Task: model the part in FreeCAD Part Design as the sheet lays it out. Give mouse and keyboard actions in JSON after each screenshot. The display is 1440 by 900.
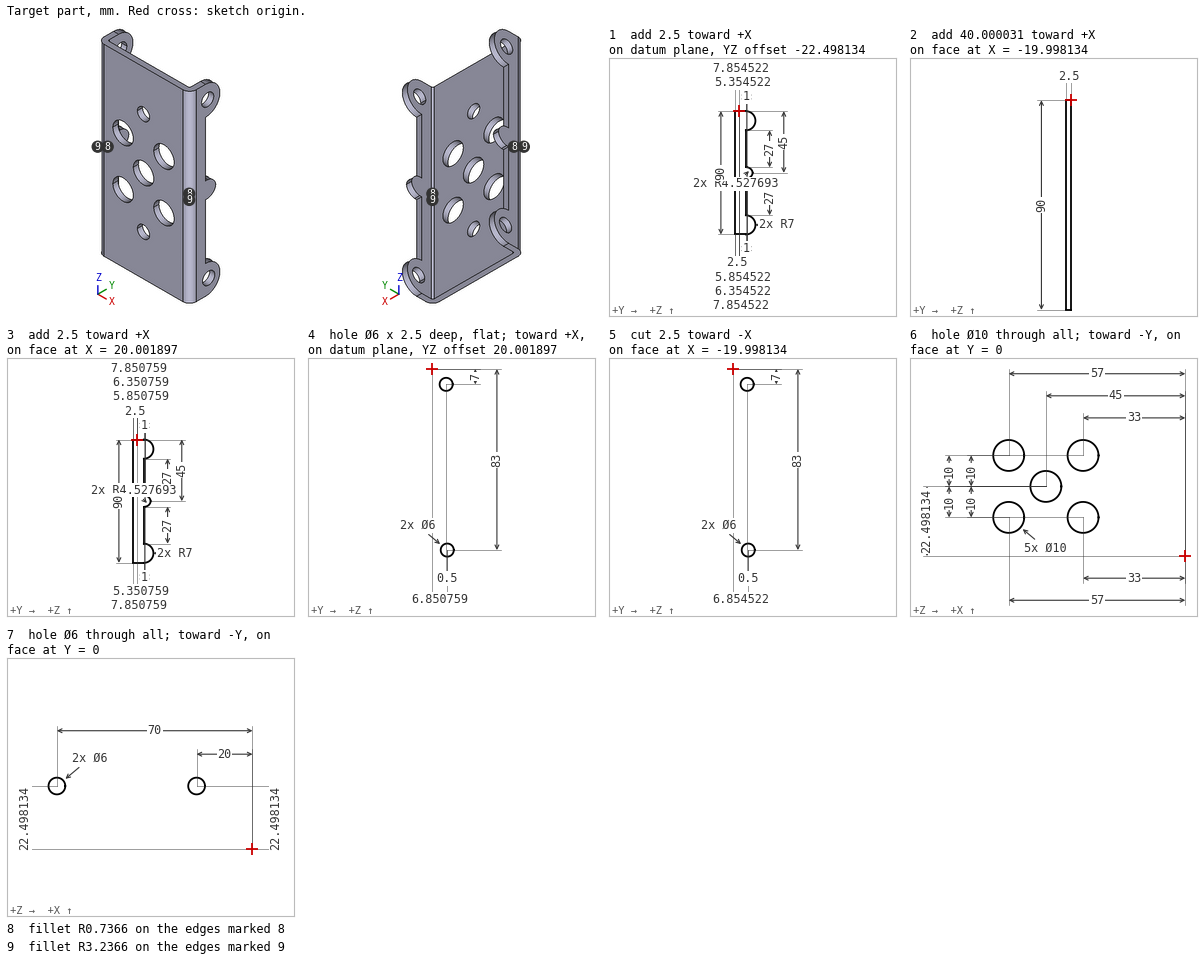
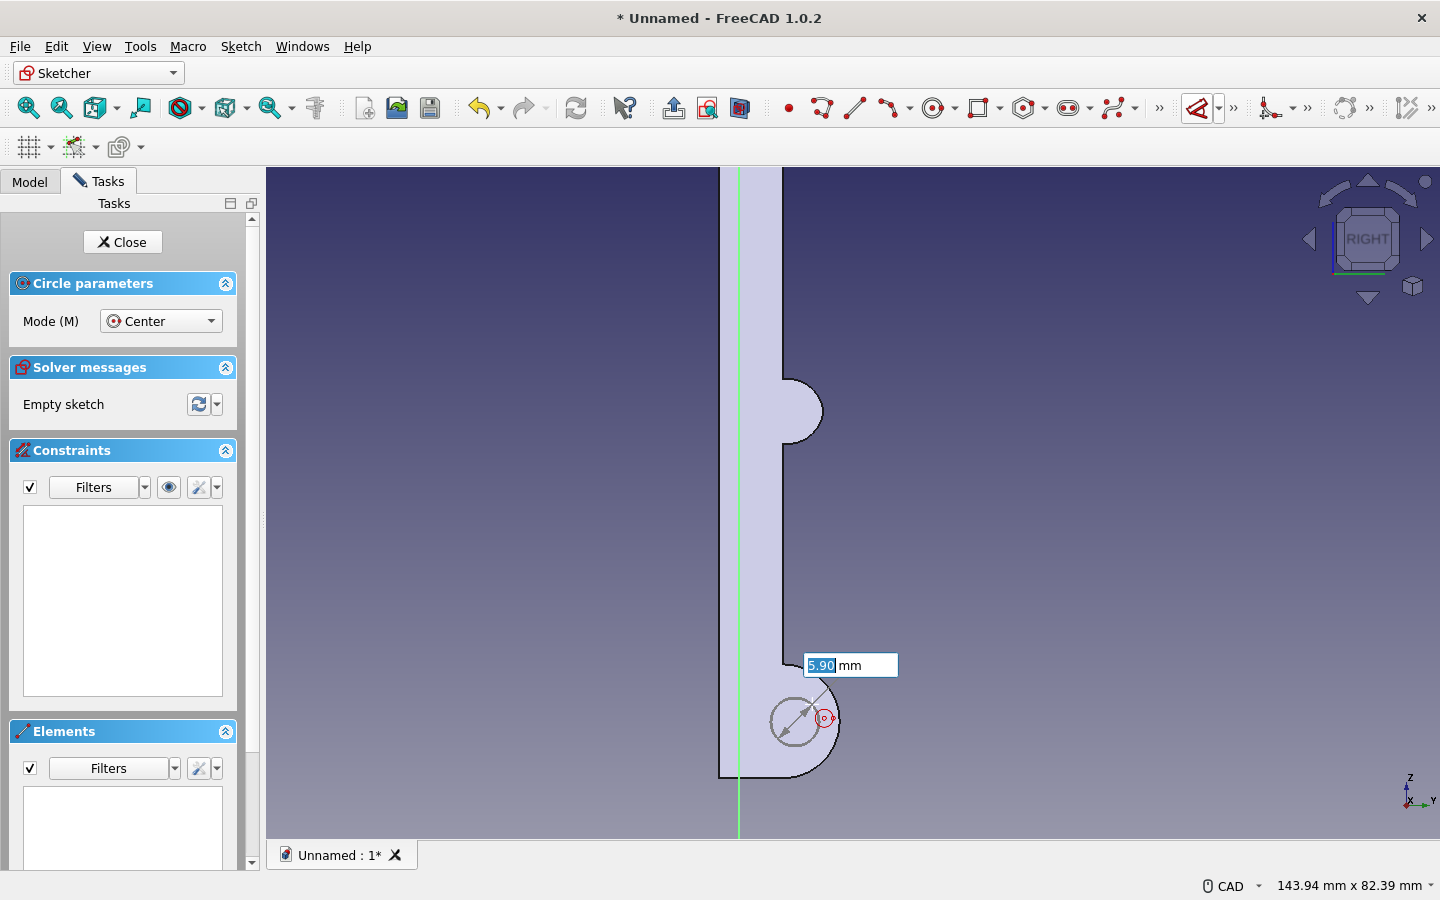
{"action": "type", "text": "6"}
{"action": "key", "text": "Return"}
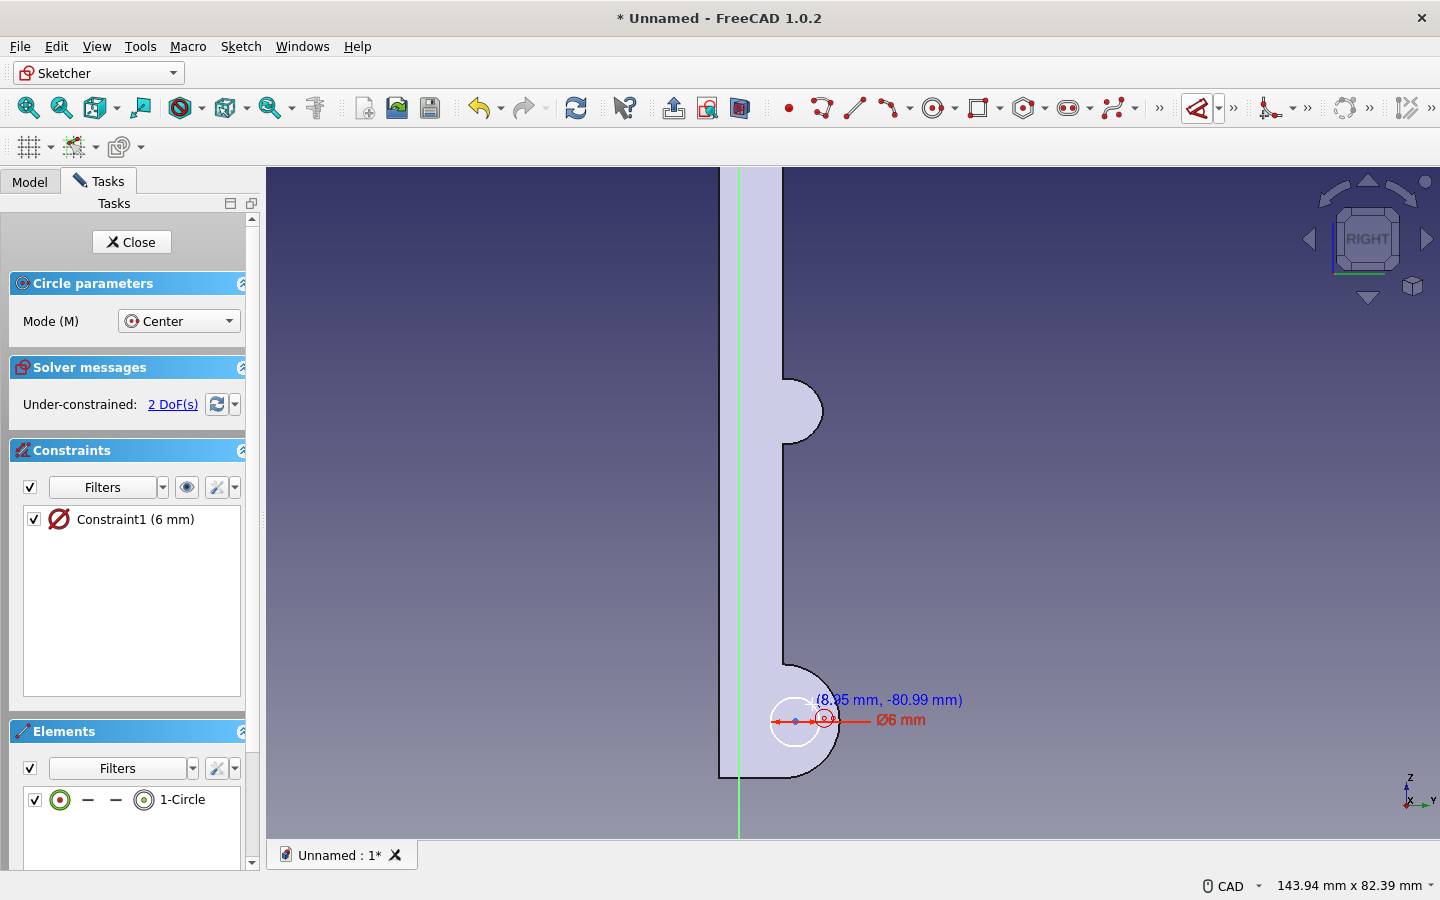
{"action": "scroll", "coordinate": [795, 722], "scroll_direction": "down", "scroll_amount": 2}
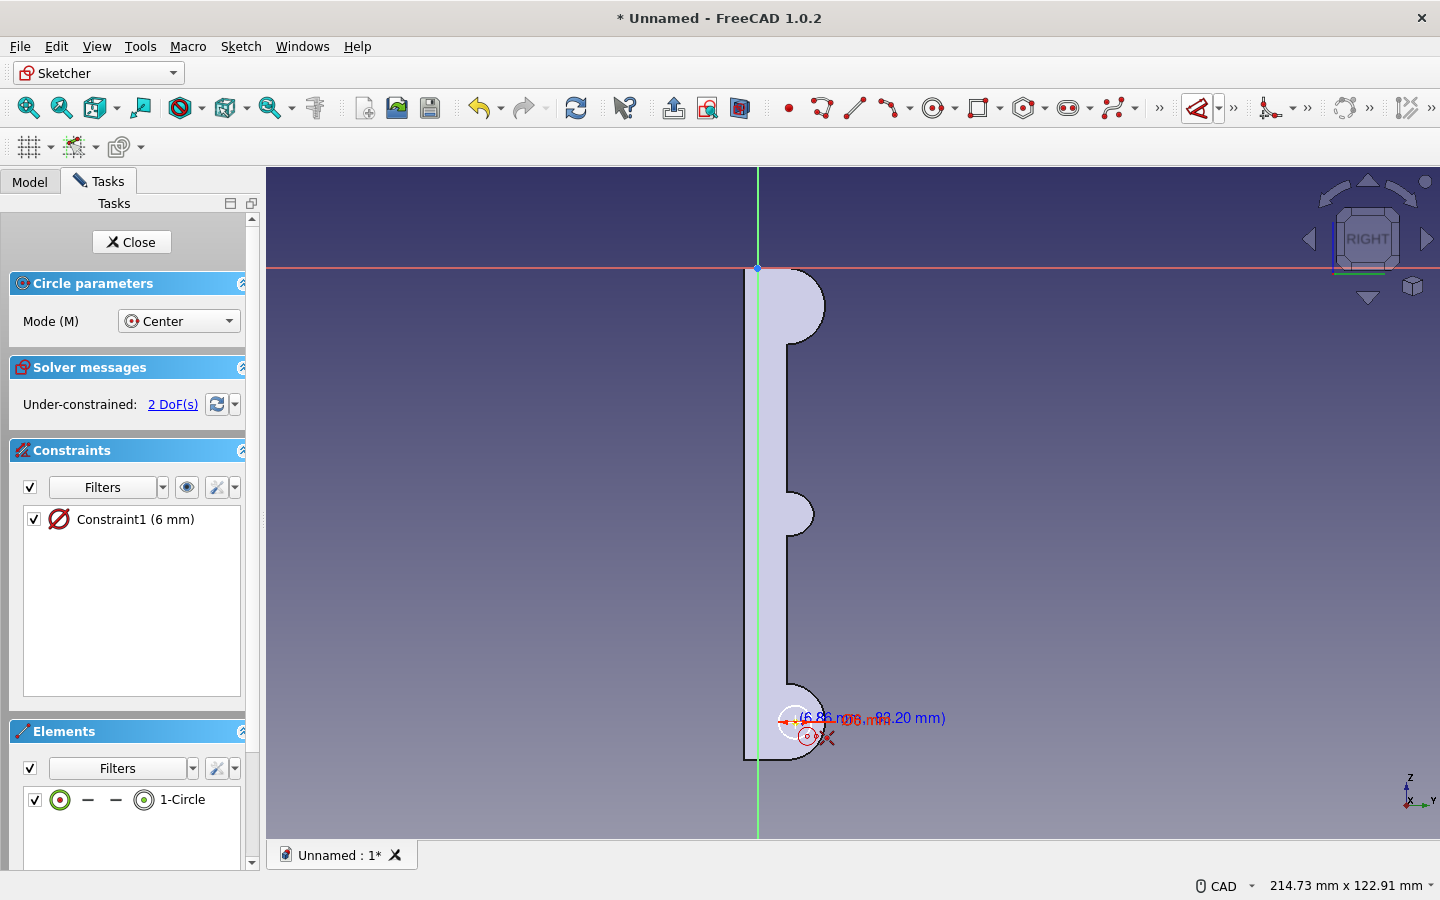
{"action": "scroll", "coordinate": [792, 306], "scroll_direction": "up", "scroll_amount": 2}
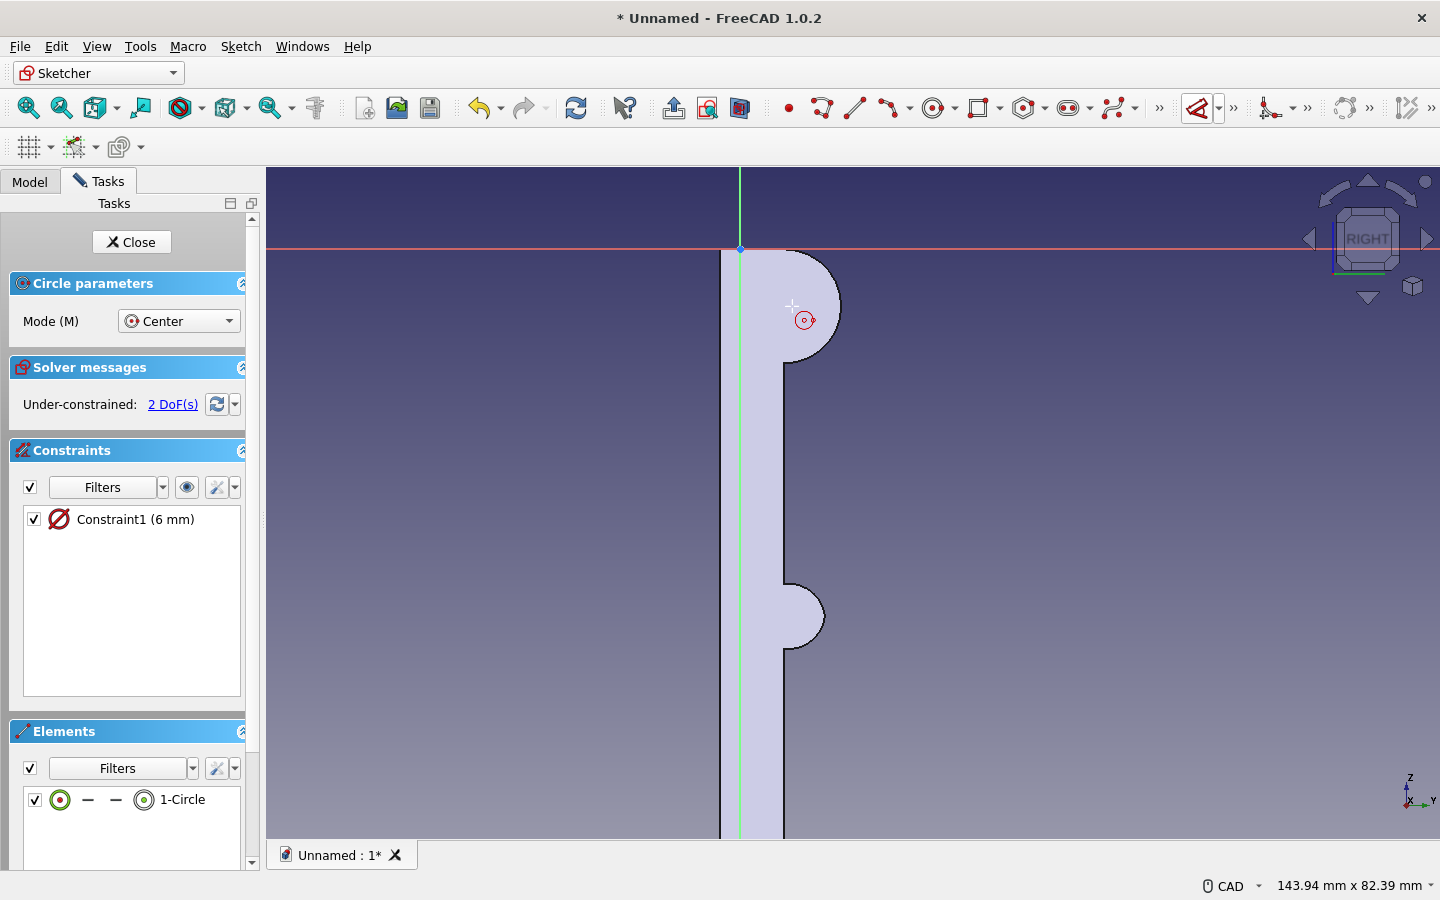
{"action": "left_click", "coordinate": [792, 306]}
{"action": "mouse_move", "coordinate": [810, 289]}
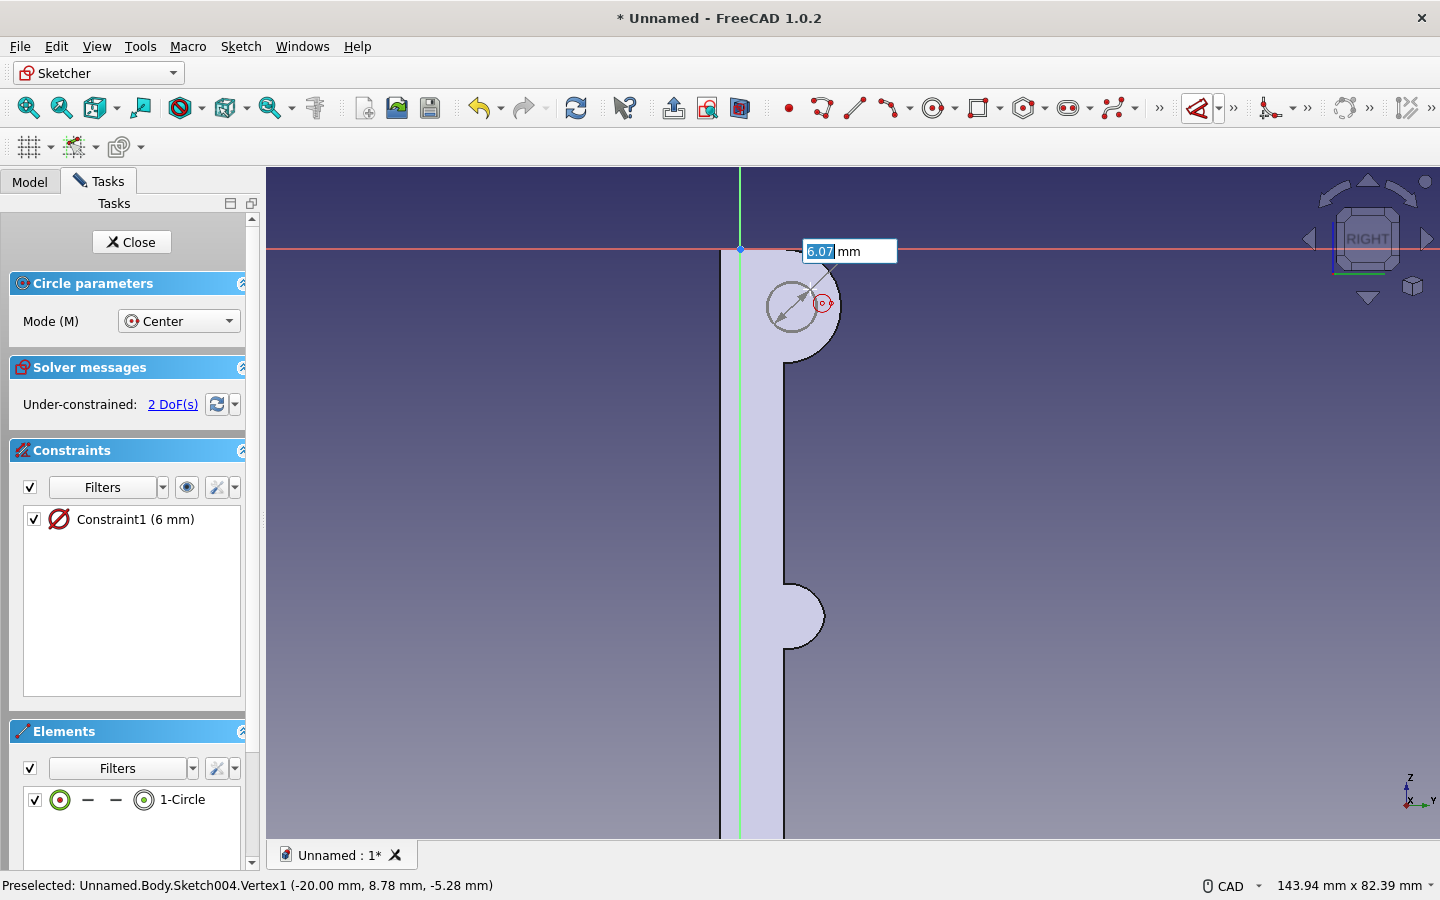
{"action": "type", "text": "6"}
{"action": "key", "text": "Return"}
{"action": "key", "text": "Escape"}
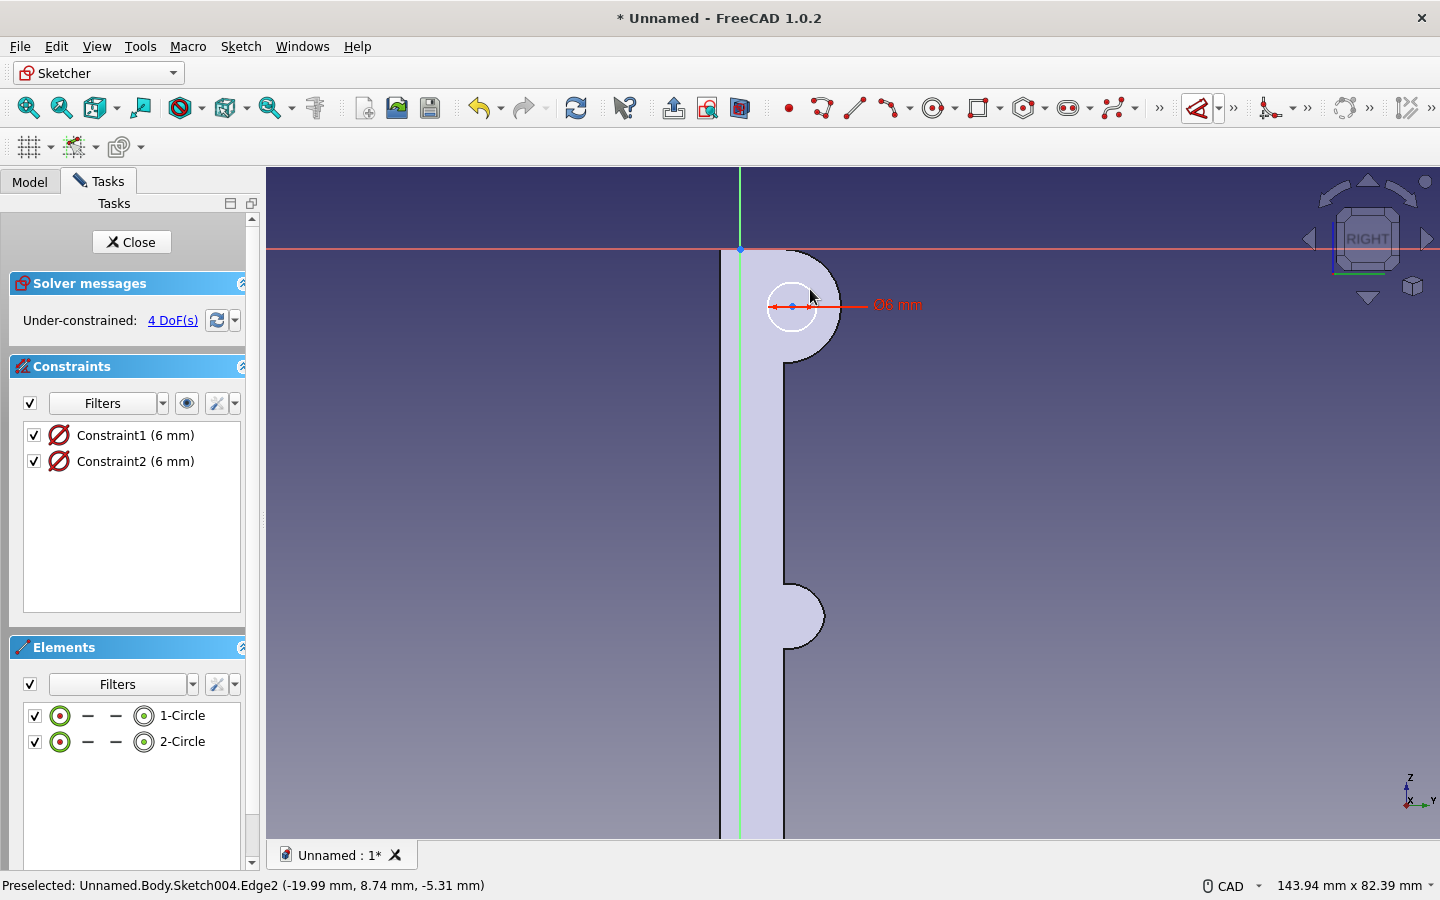
{"action": "left_click", "coordinate": [792, 307]}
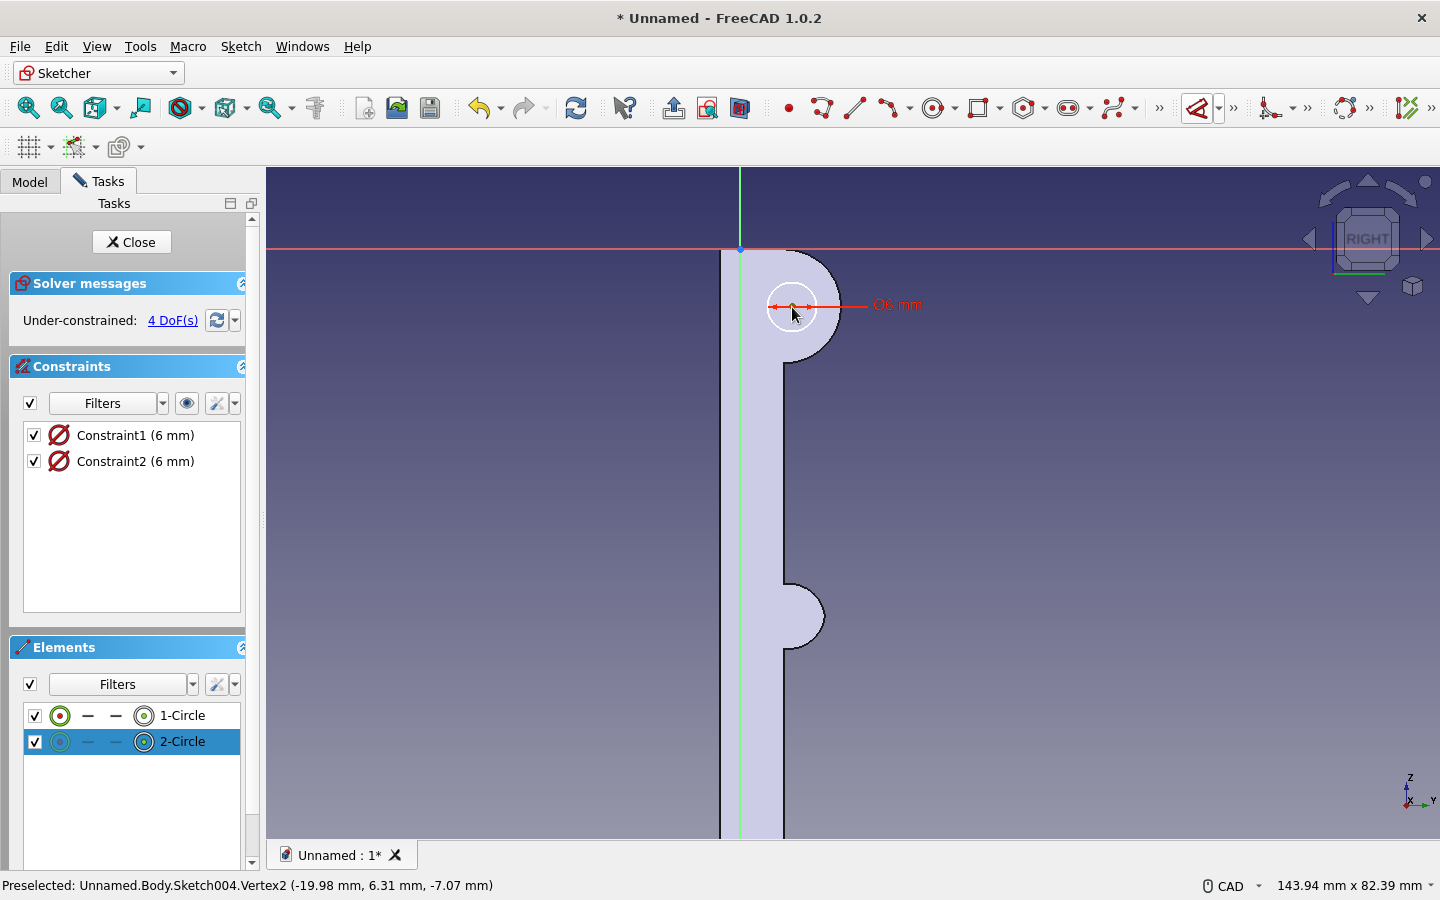
{"action": "left_click", "coordinate": [1218, 108]}